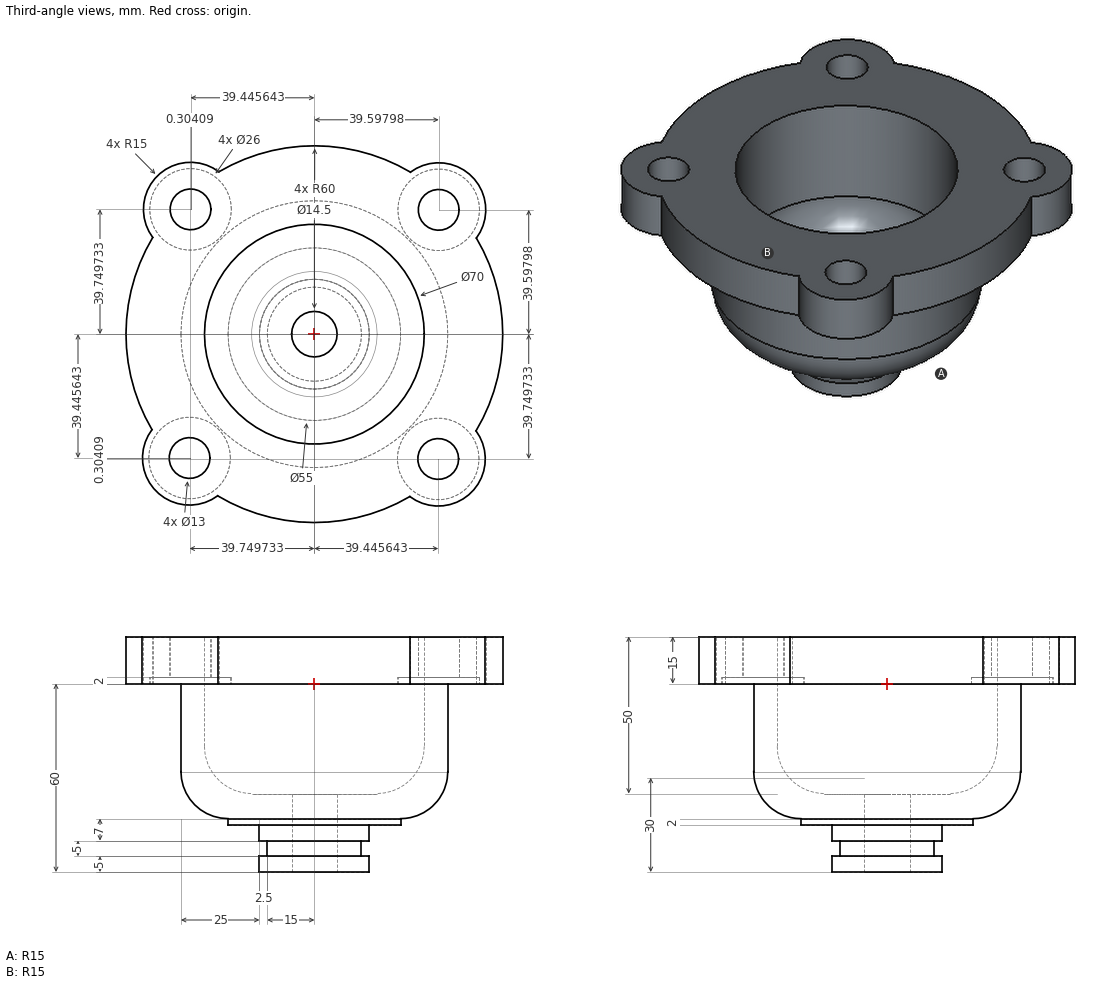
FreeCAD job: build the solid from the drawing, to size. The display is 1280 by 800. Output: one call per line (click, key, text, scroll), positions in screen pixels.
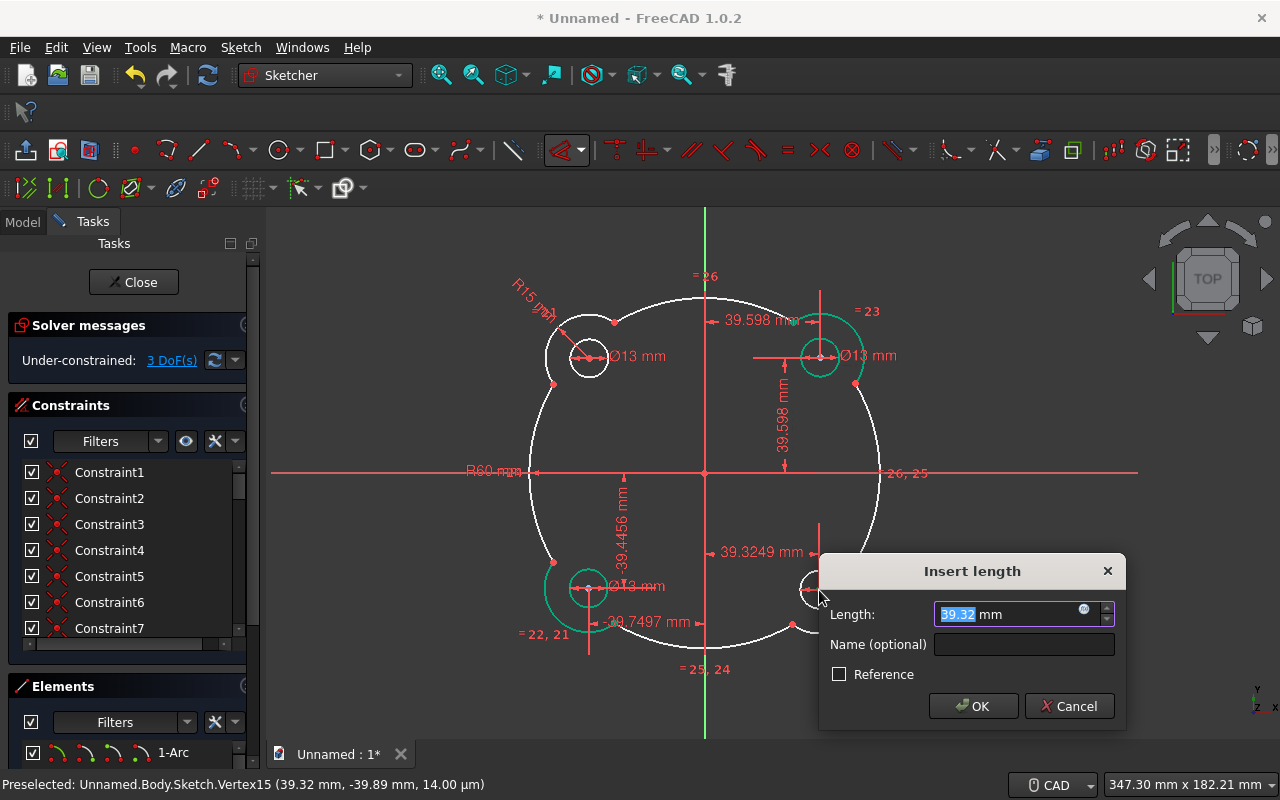
text(39.445643)
key(Return)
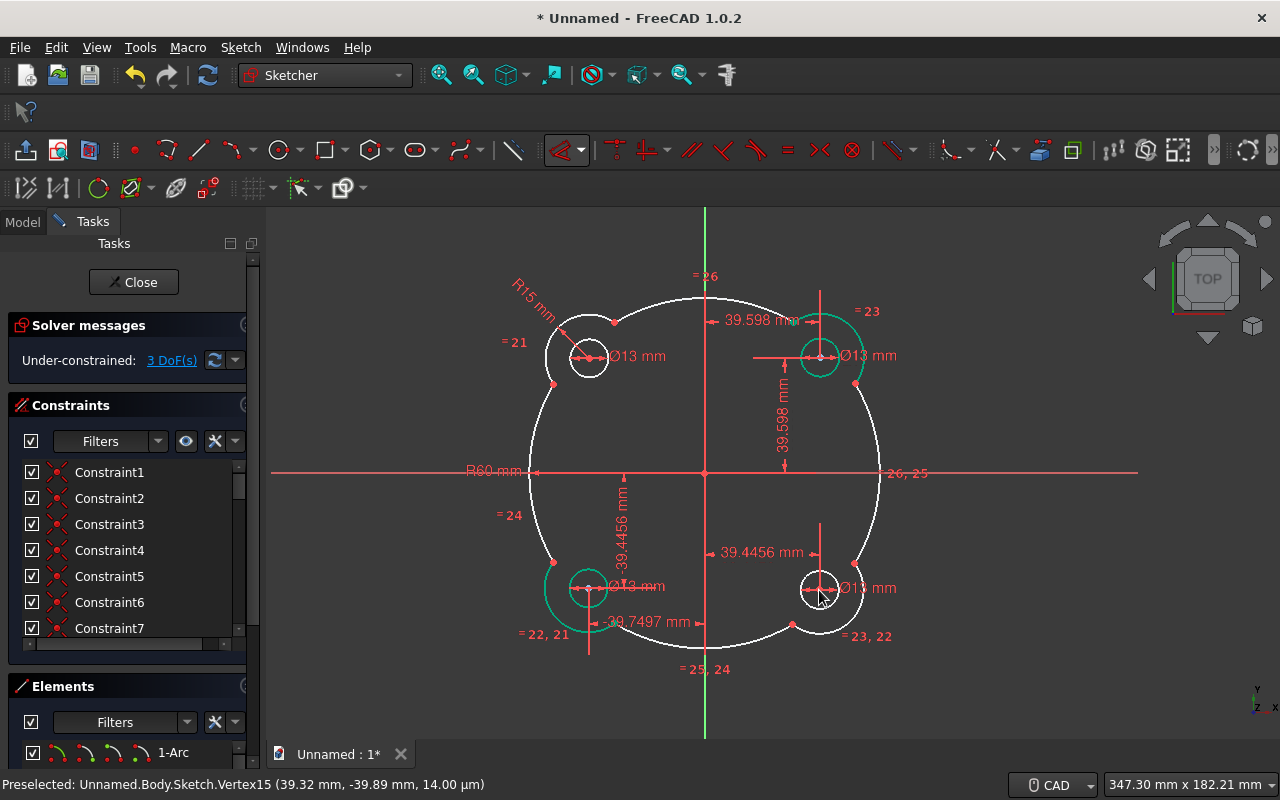
click(820, 590)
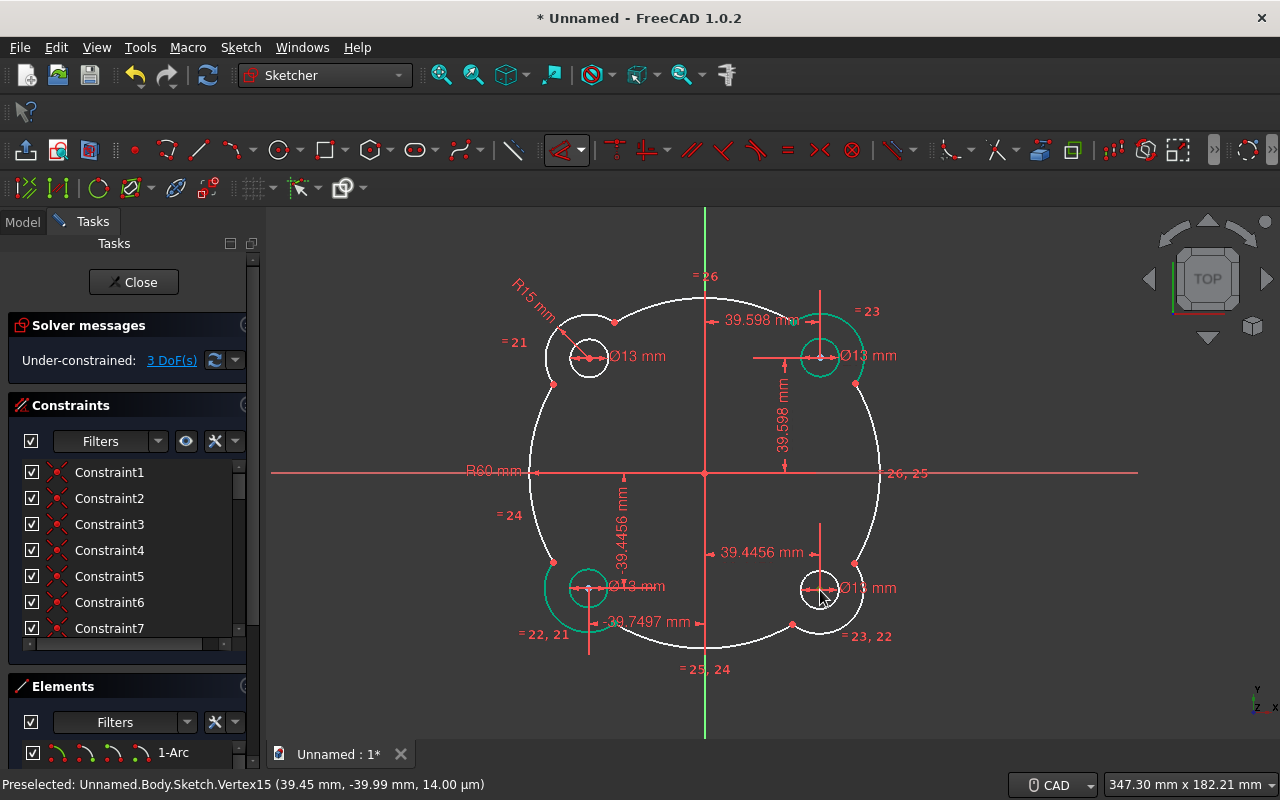
key(i)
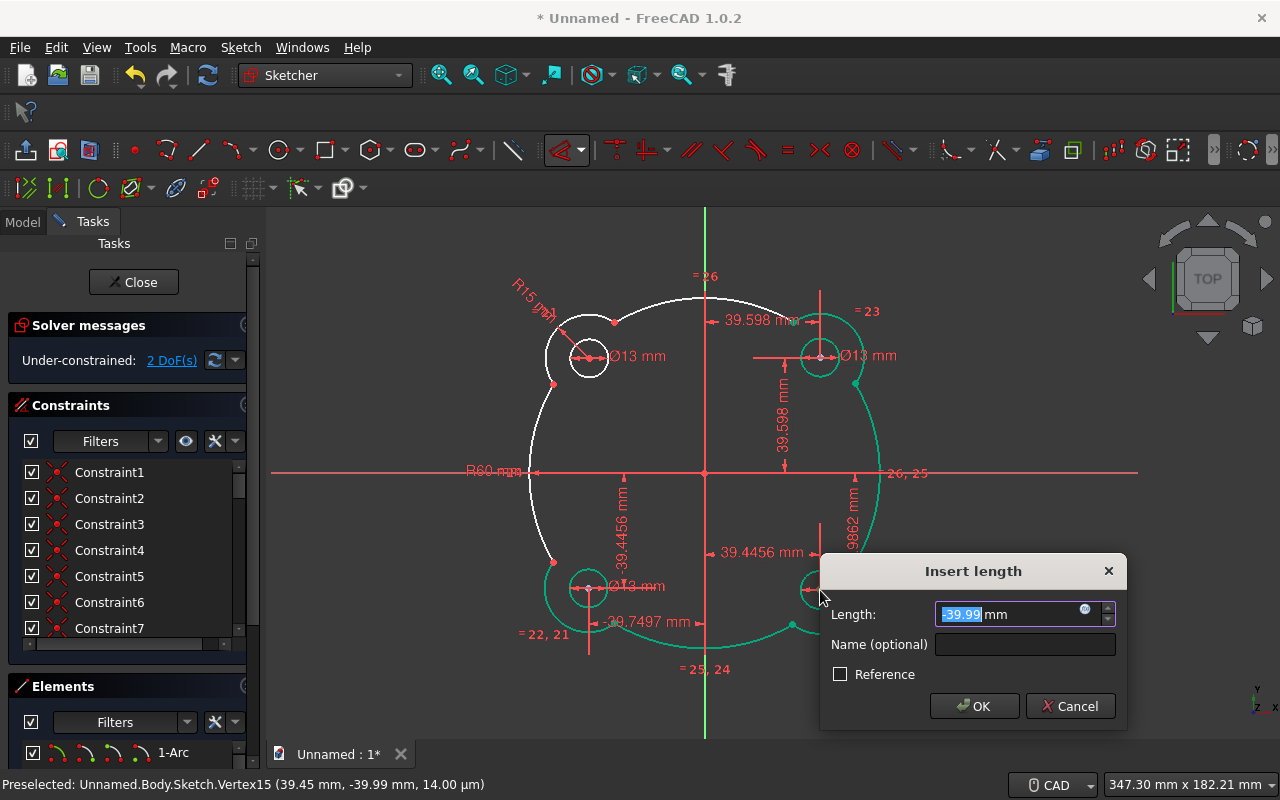
text(-39.749733)
key(Return)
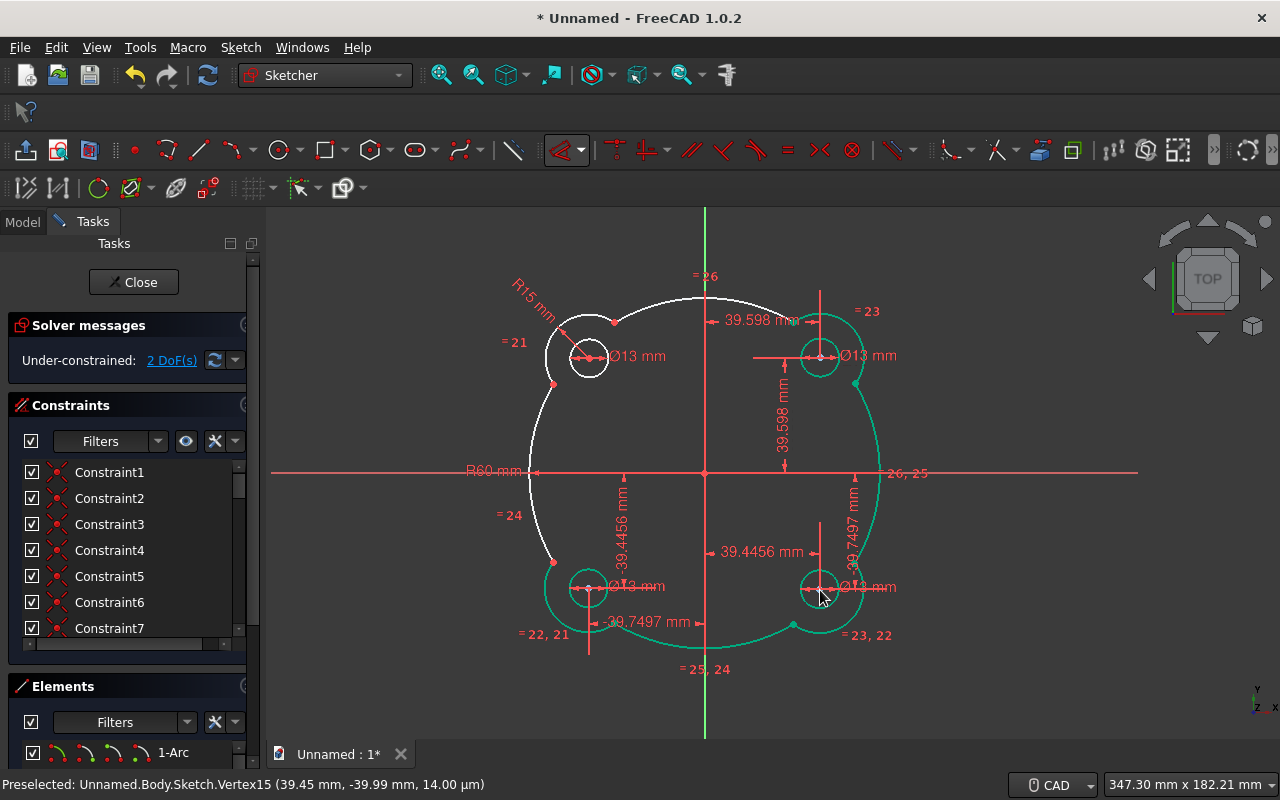
click(589, 358)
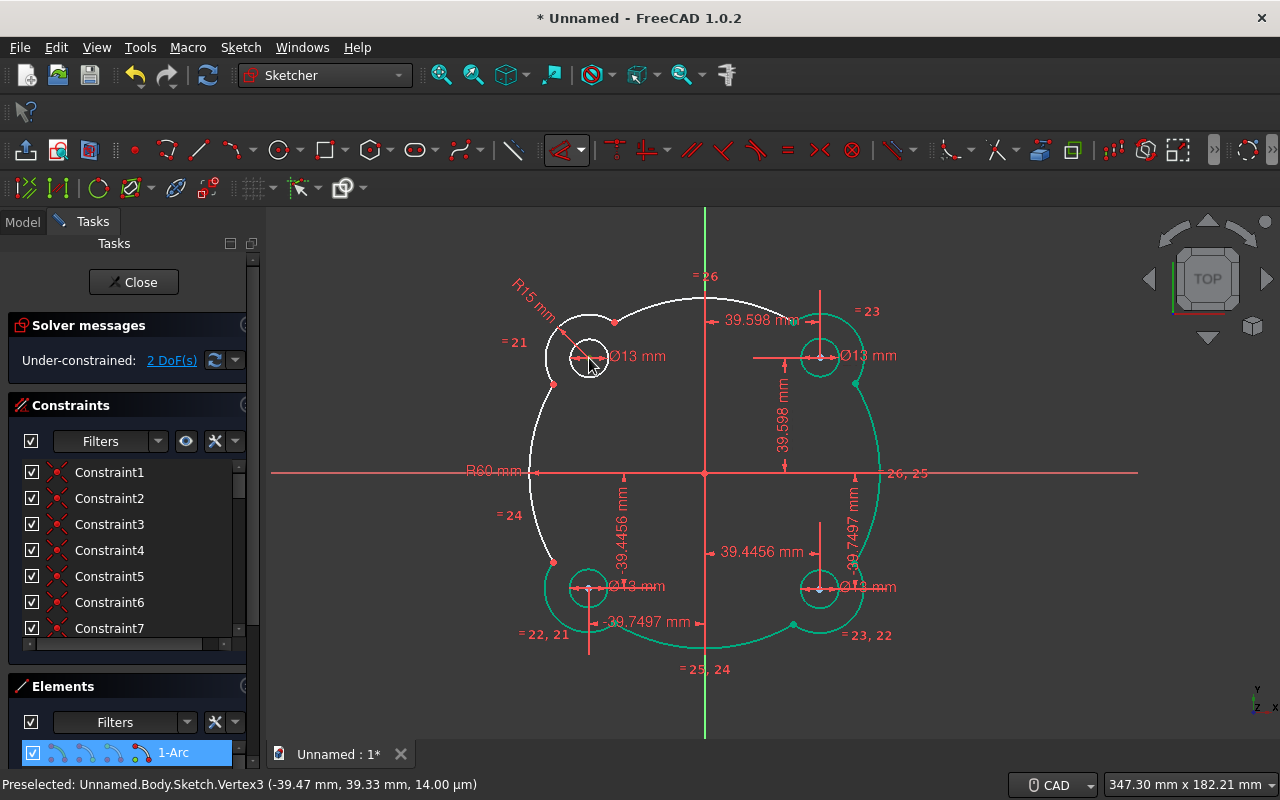
click(584, 150)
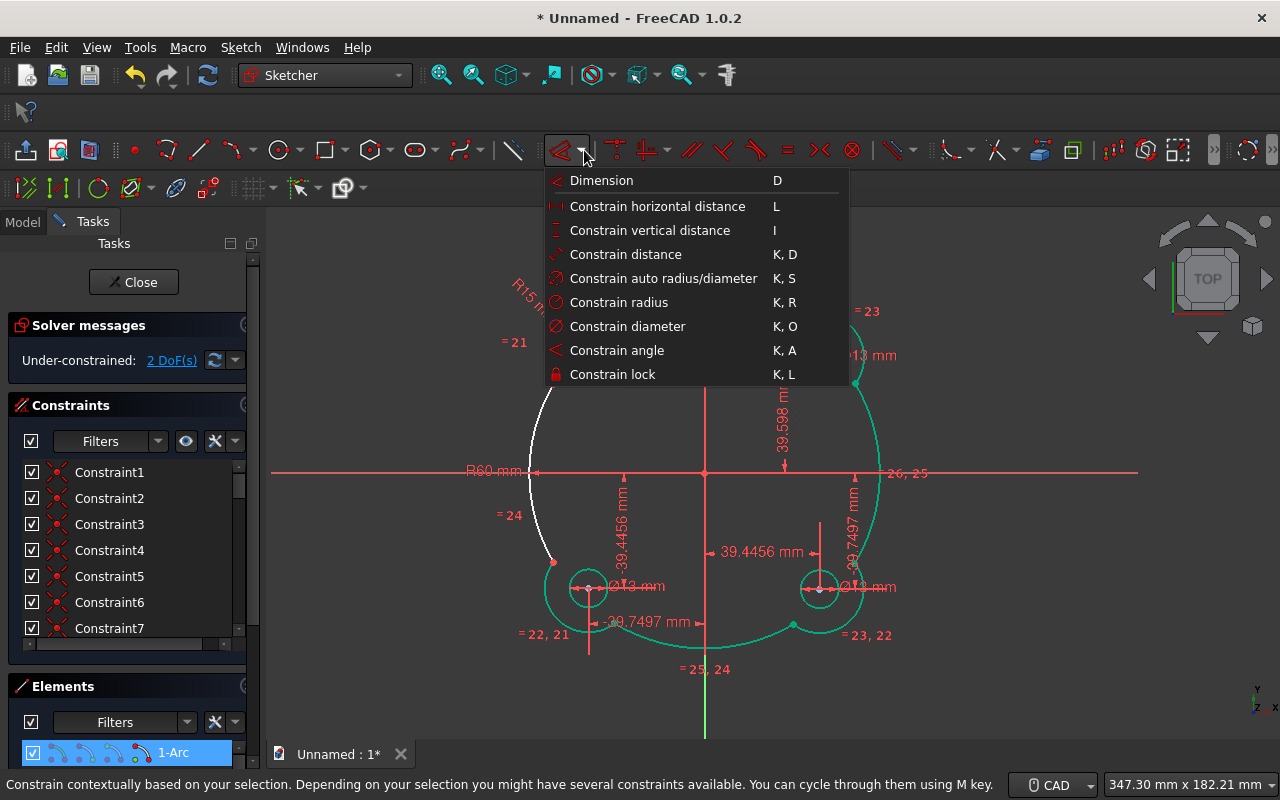
click(697, 206)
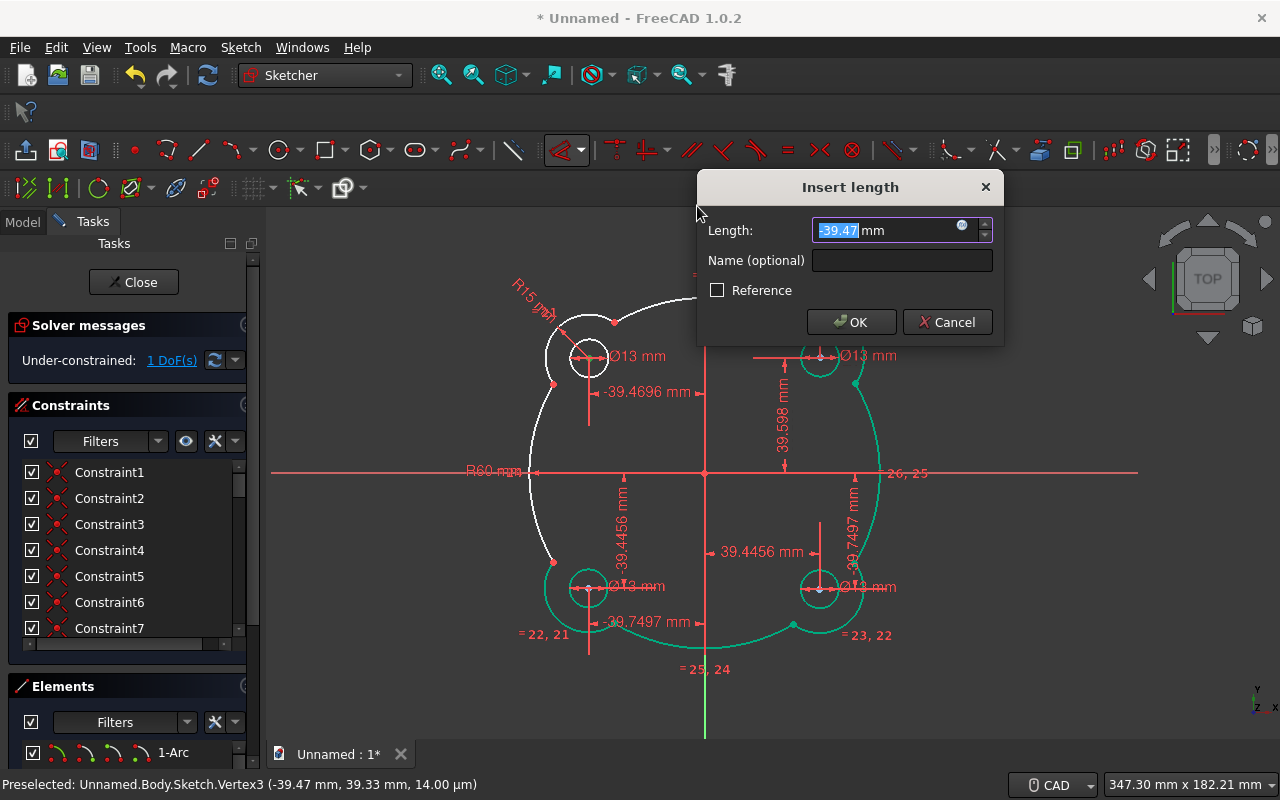
text(-39.445643)
key(Return)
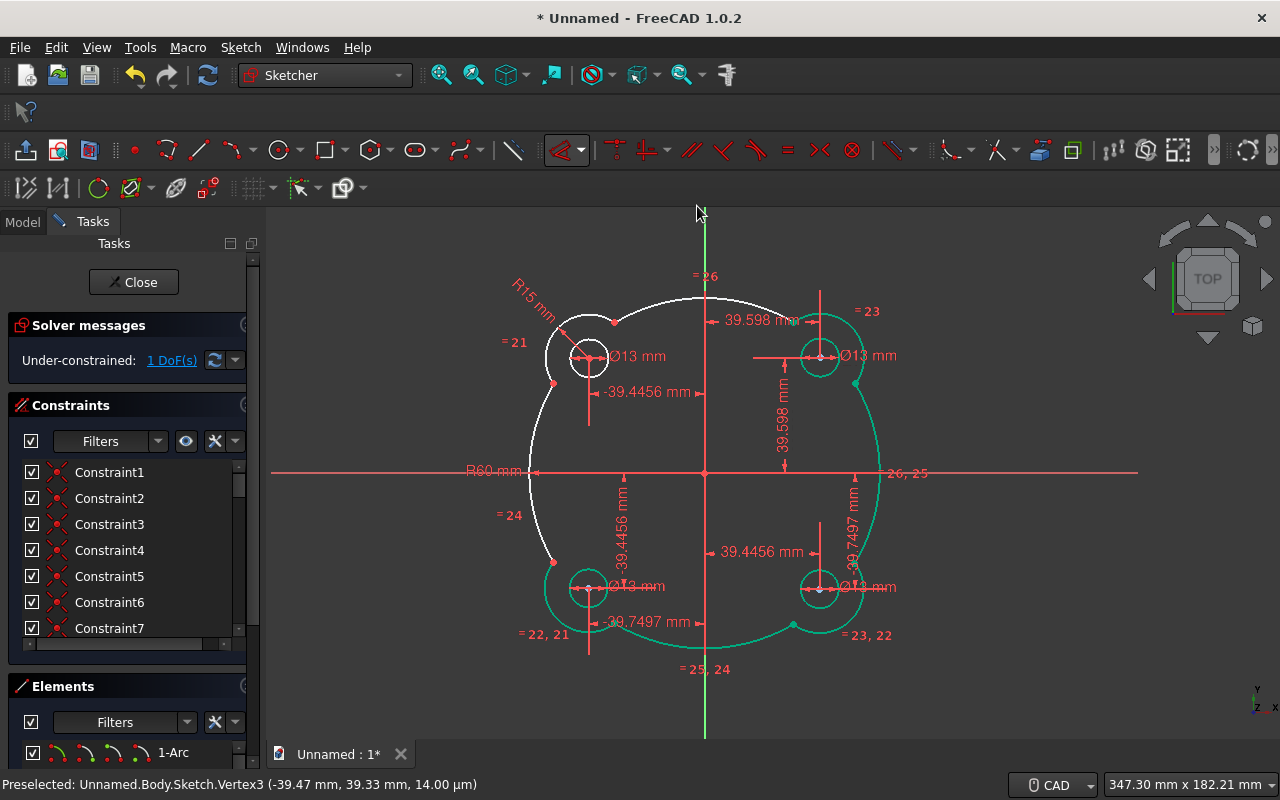
click(589, 358)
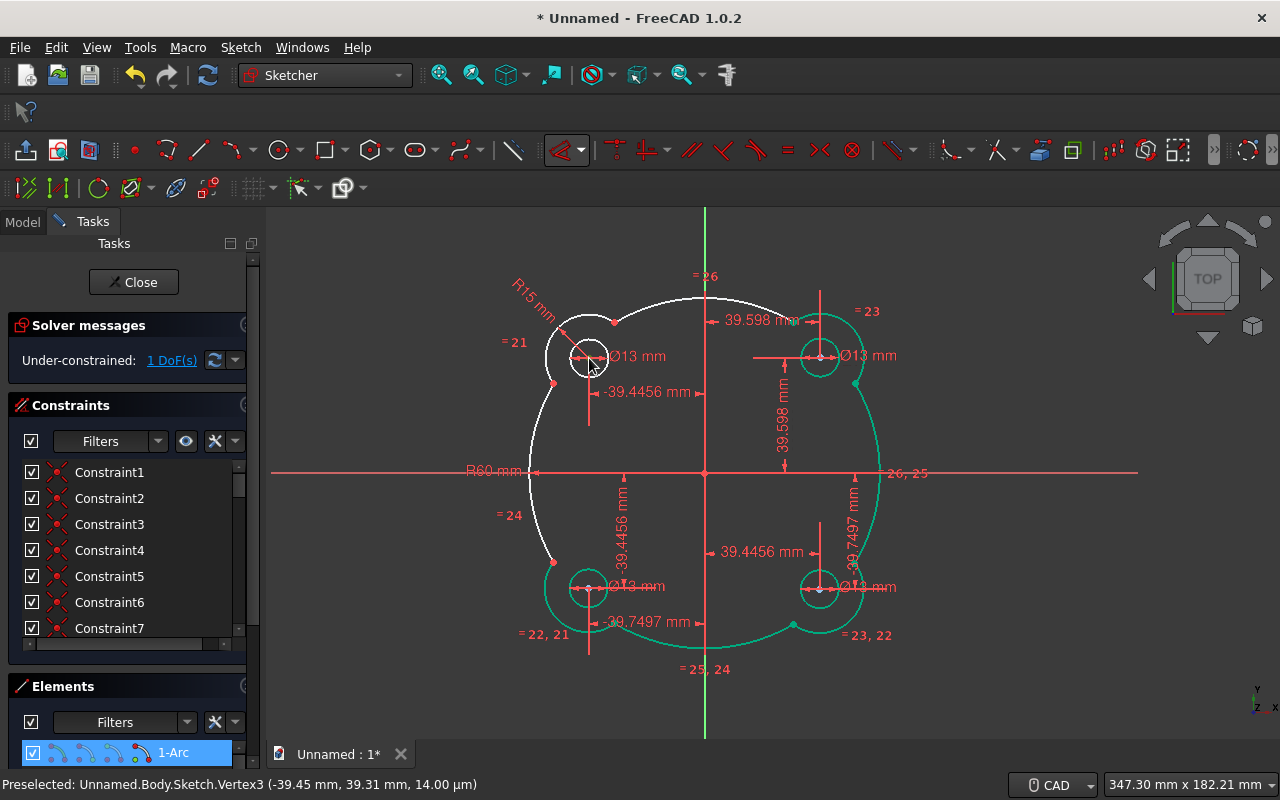
click(584, 150)